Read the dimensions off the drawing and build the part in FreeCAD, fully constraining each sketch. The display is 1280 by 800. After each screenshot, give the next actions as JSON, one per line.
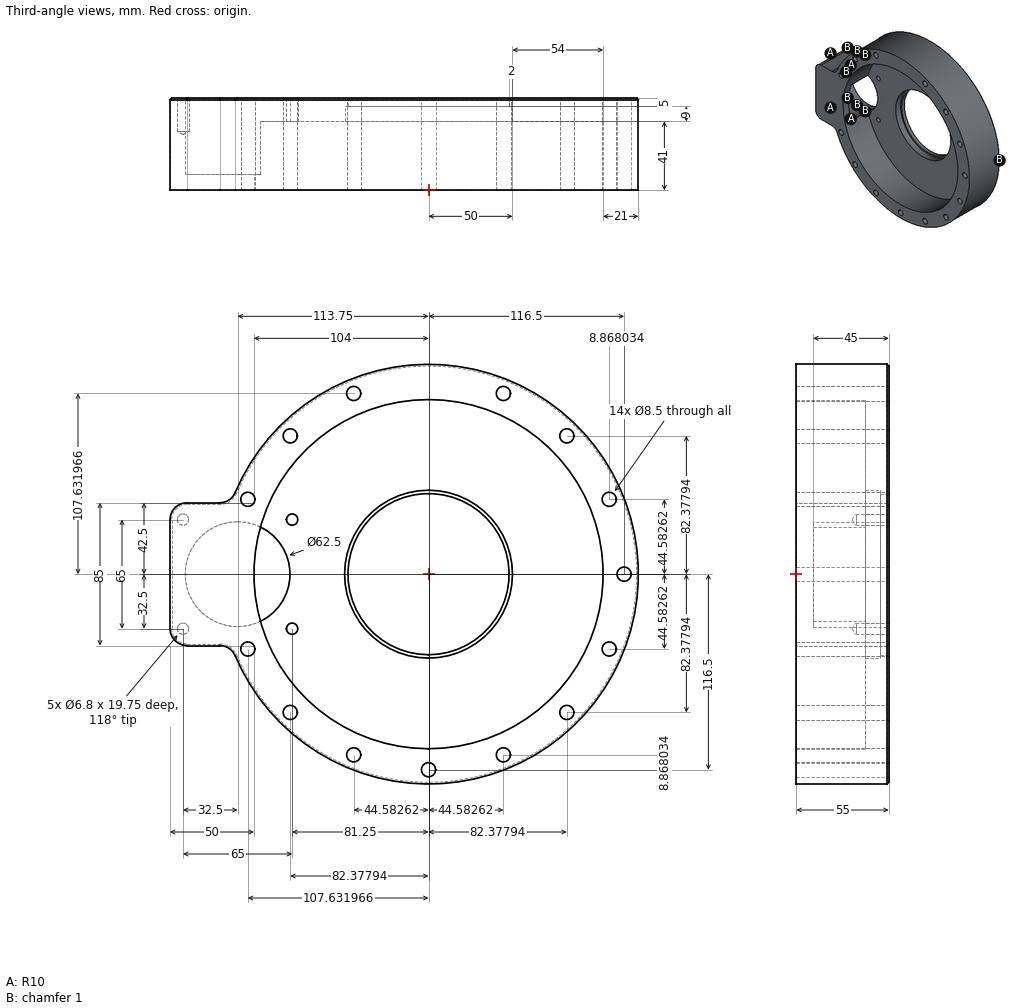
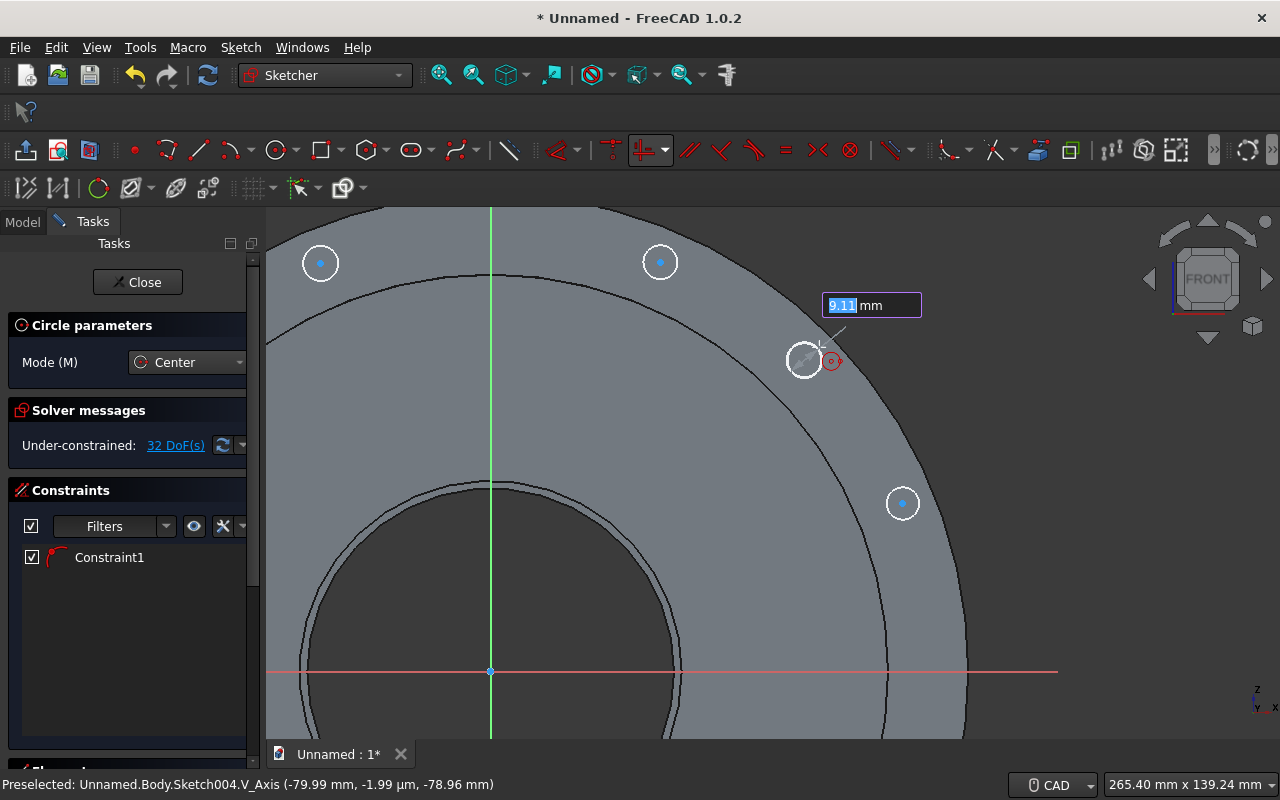
{"action": "left_click", "coordinate": [817, 346]}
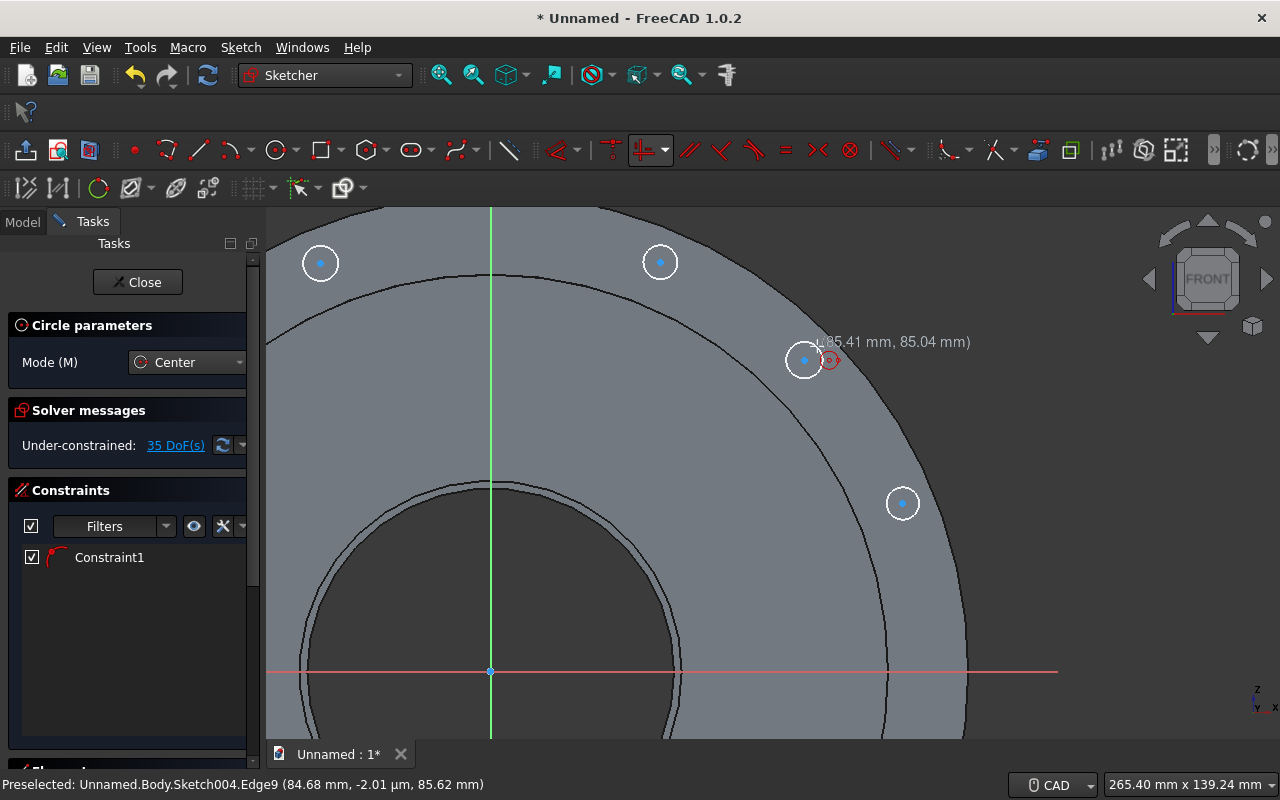
{"action": "scroll", "coordinate": [819, 347], "scroll_direction": "down", "scroll_amount": 5}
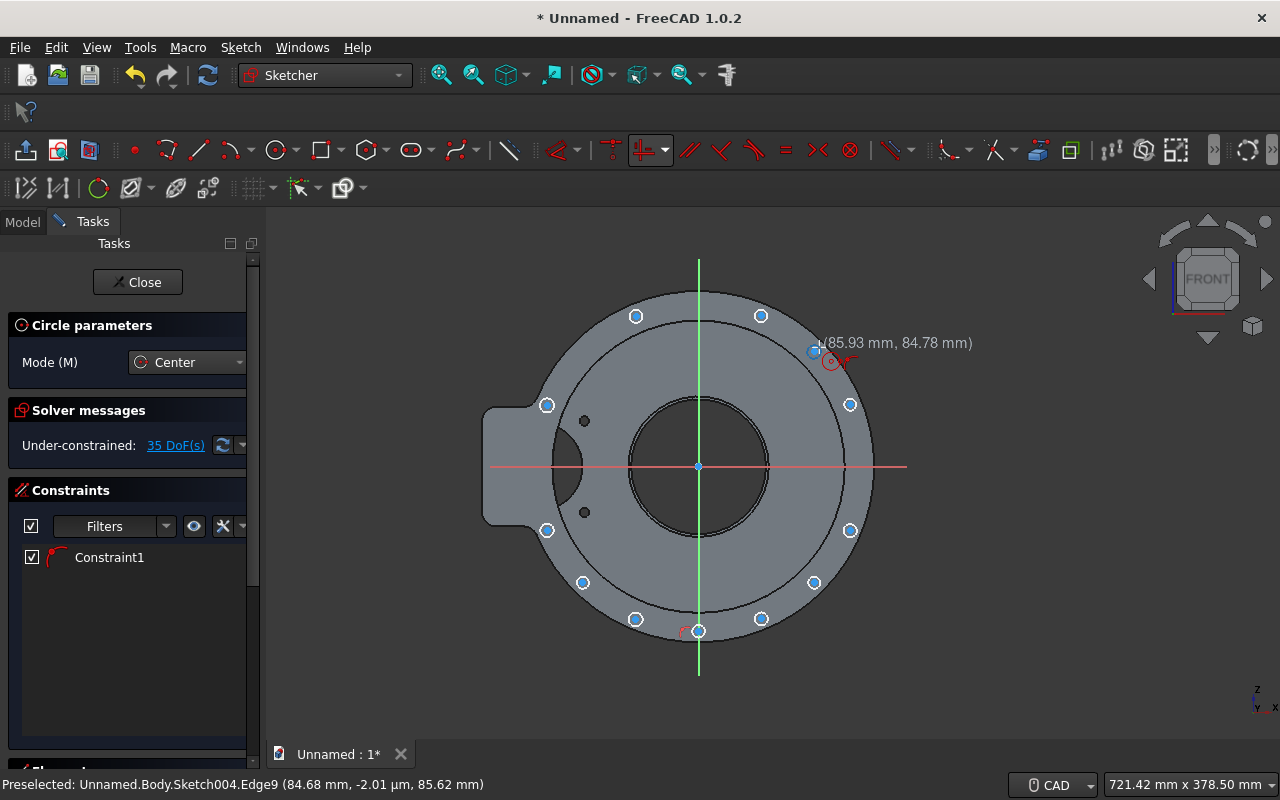
{"action": "scroll", "coordinate": [583, 351], "scroll_direction": "up", "scroll_amount": 7}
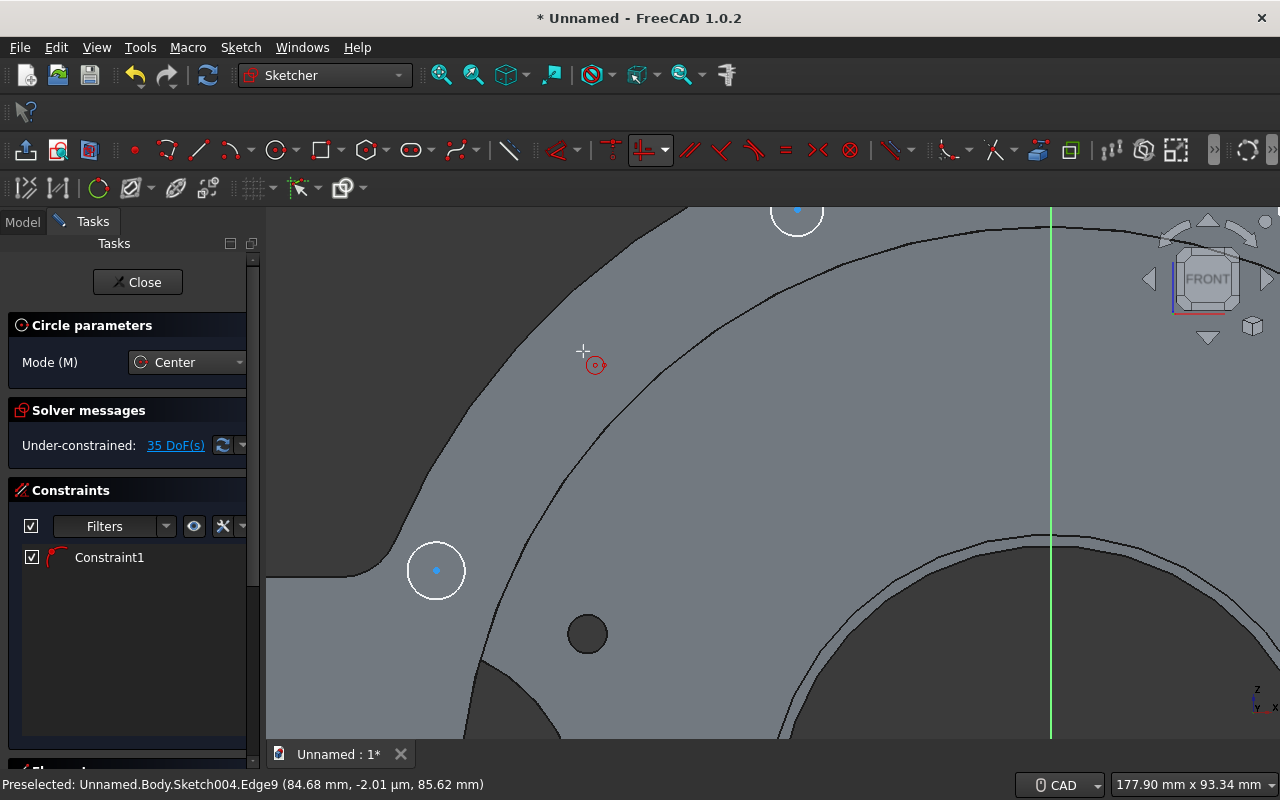
{"action": "scroll", "coordinate": [583, 351], "scroll_direction": "down", "scroll_amount": 7}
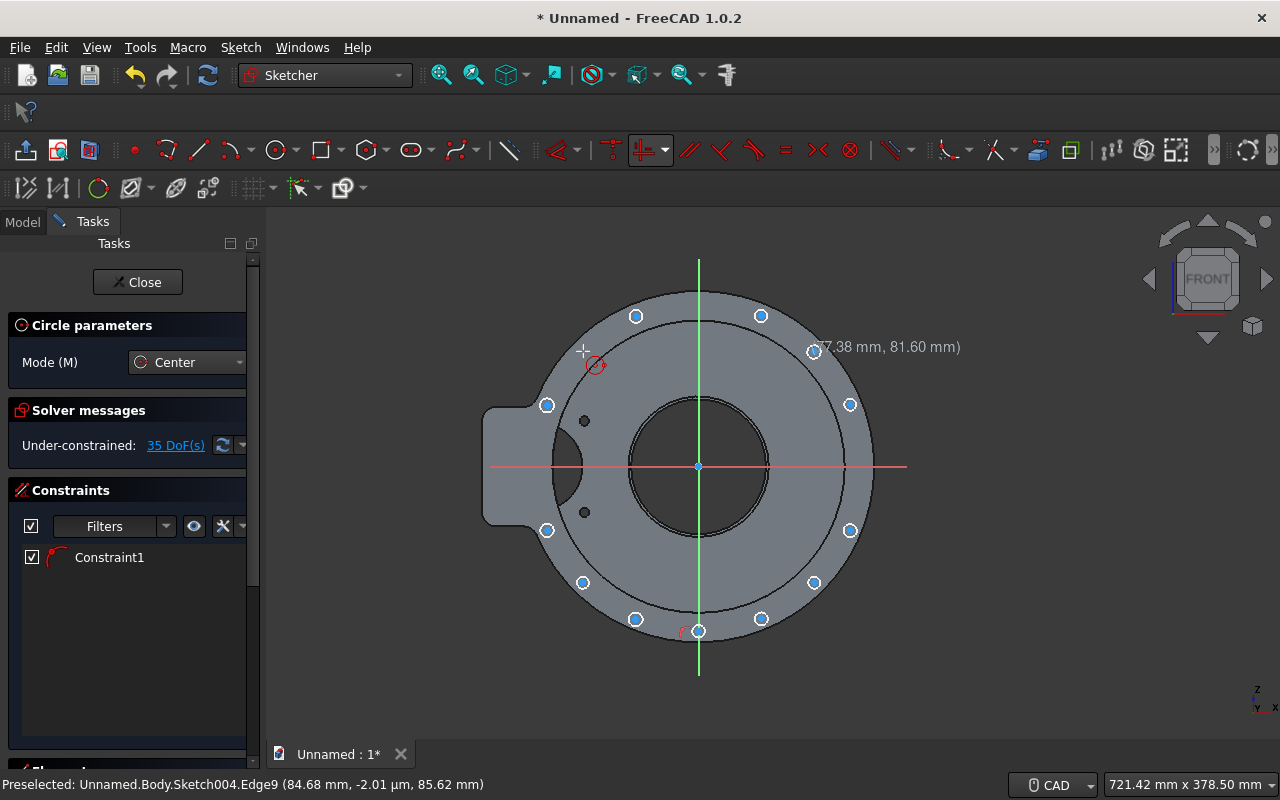
{"action": "left_click", "coordinate": [583, 351]}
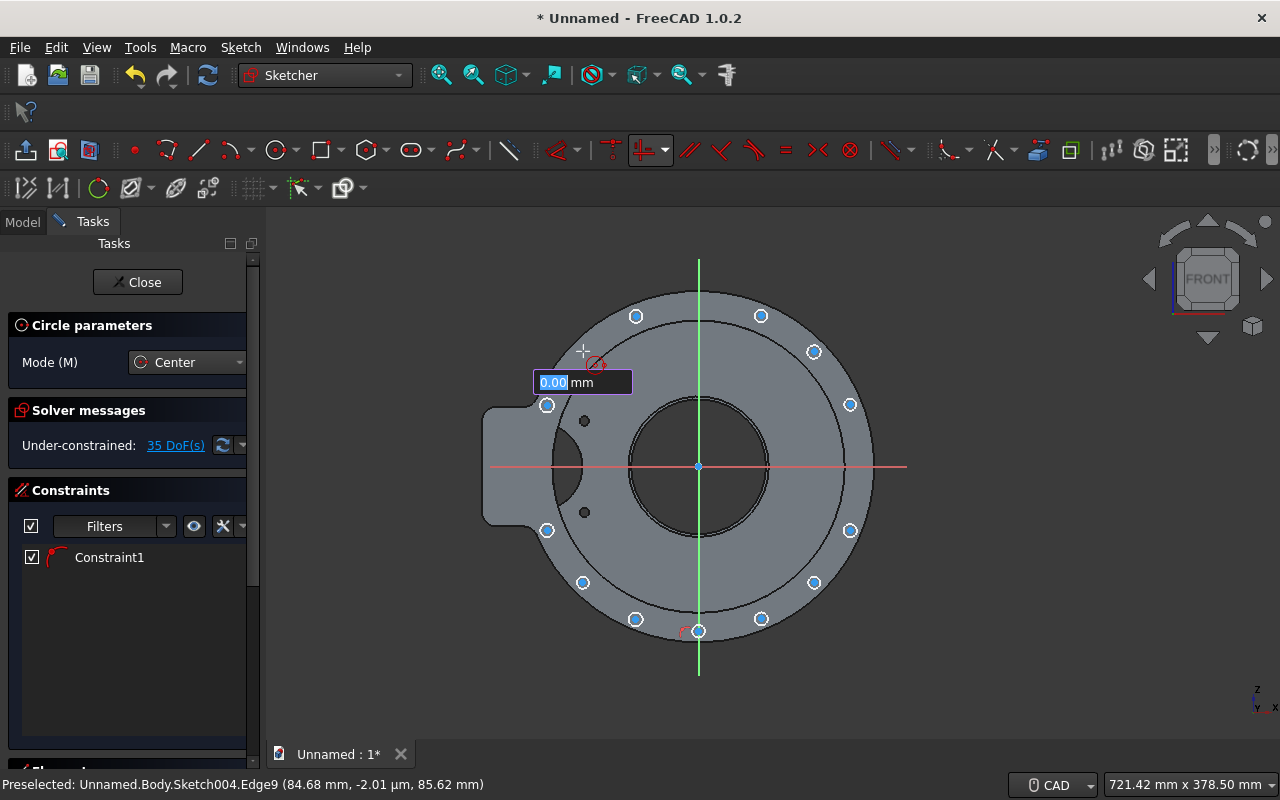
{"action": "scroll", "coordinate": [587, 347], "scroll_direction": "up", "scroll_amount": 5}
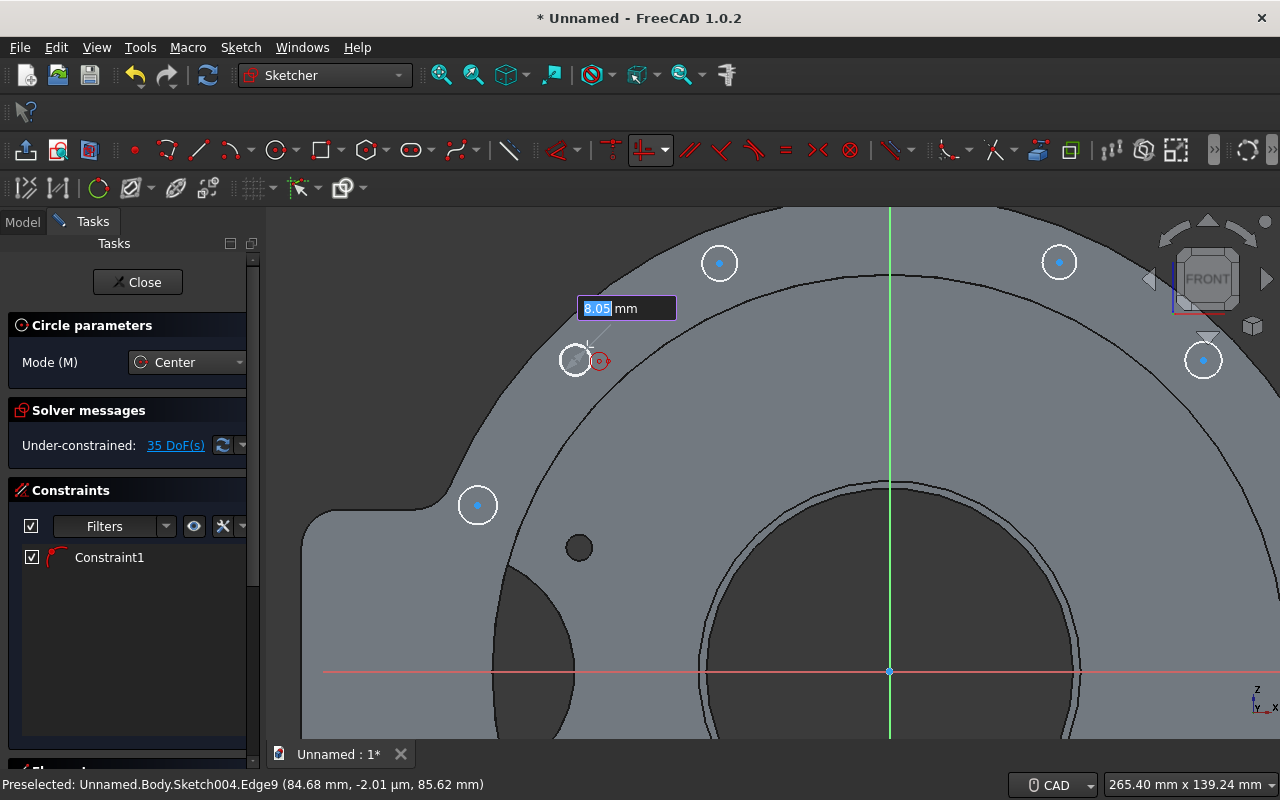
{"action": "left_click", "coordinate": [586, 346]}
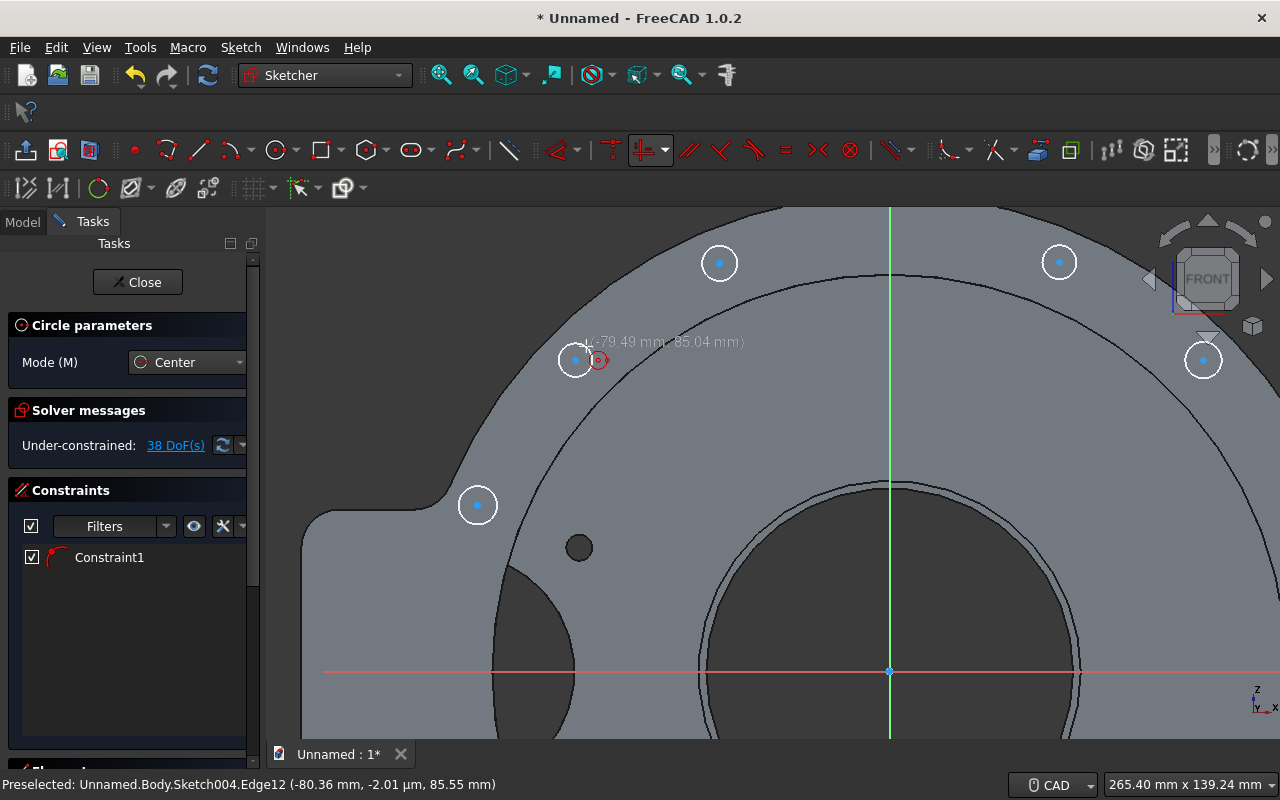
{"action": "scroll", "coordinate": [587, 347], "scroll_direction": "down", "scroll_amount": 5}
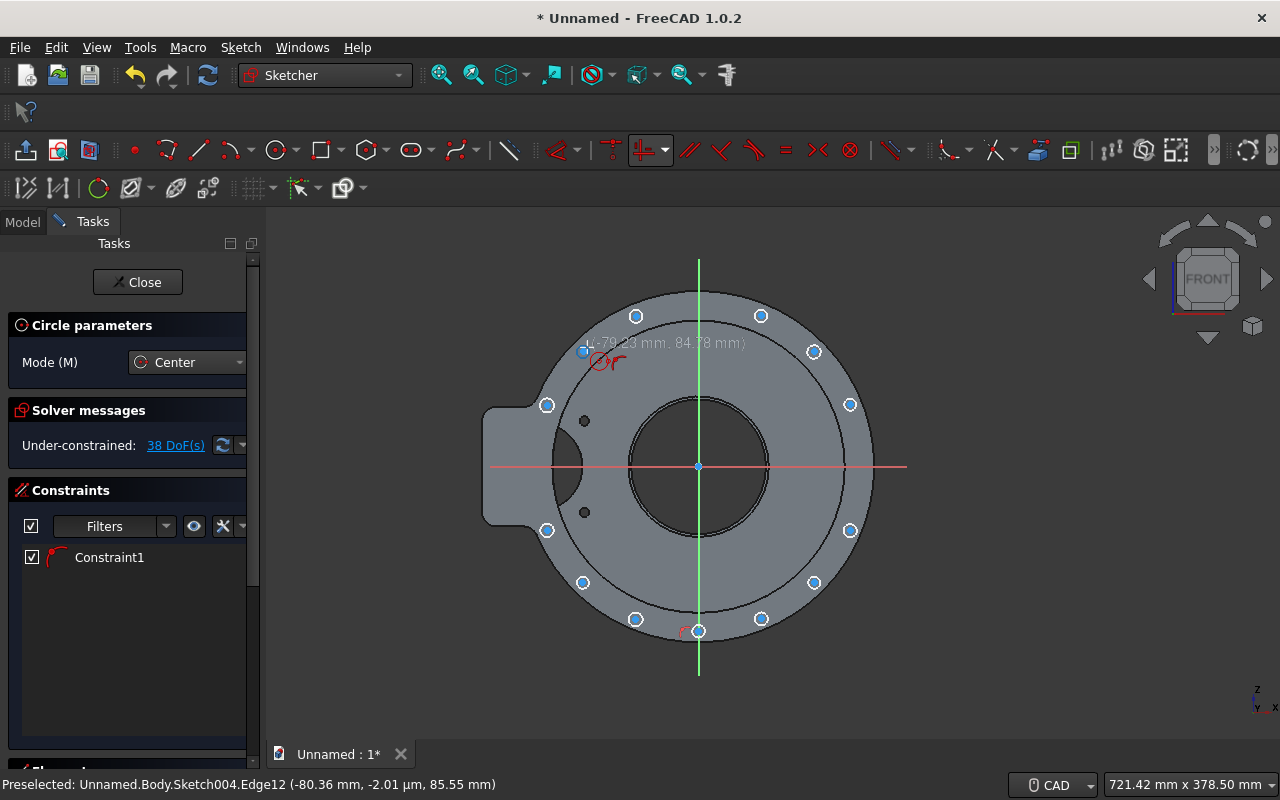
{"action": "scroll", "coordinate": [862, 467], "scroll_direction": "up", "scroll_amount": 7}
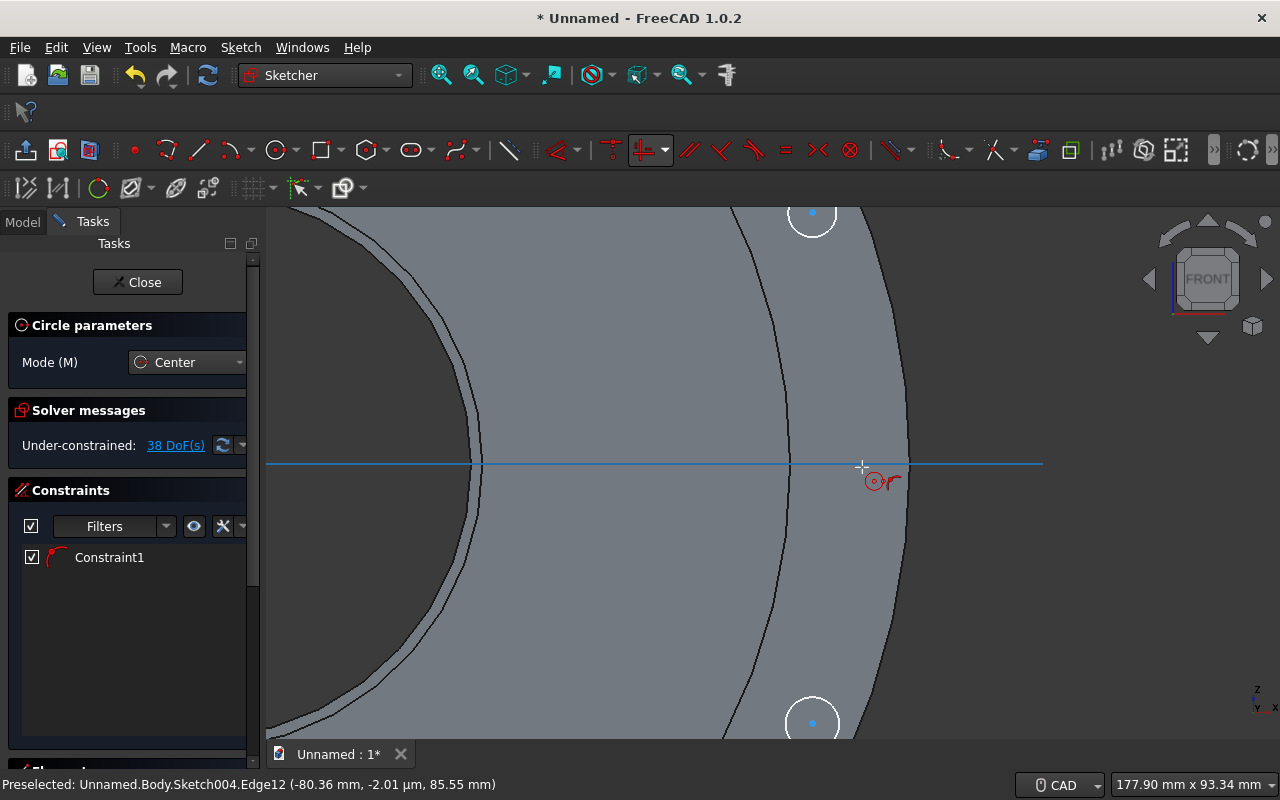
{"action": "scroll", "coordinate": [862, 468], "scroll_direction": "down", "scroll_amount": 7}